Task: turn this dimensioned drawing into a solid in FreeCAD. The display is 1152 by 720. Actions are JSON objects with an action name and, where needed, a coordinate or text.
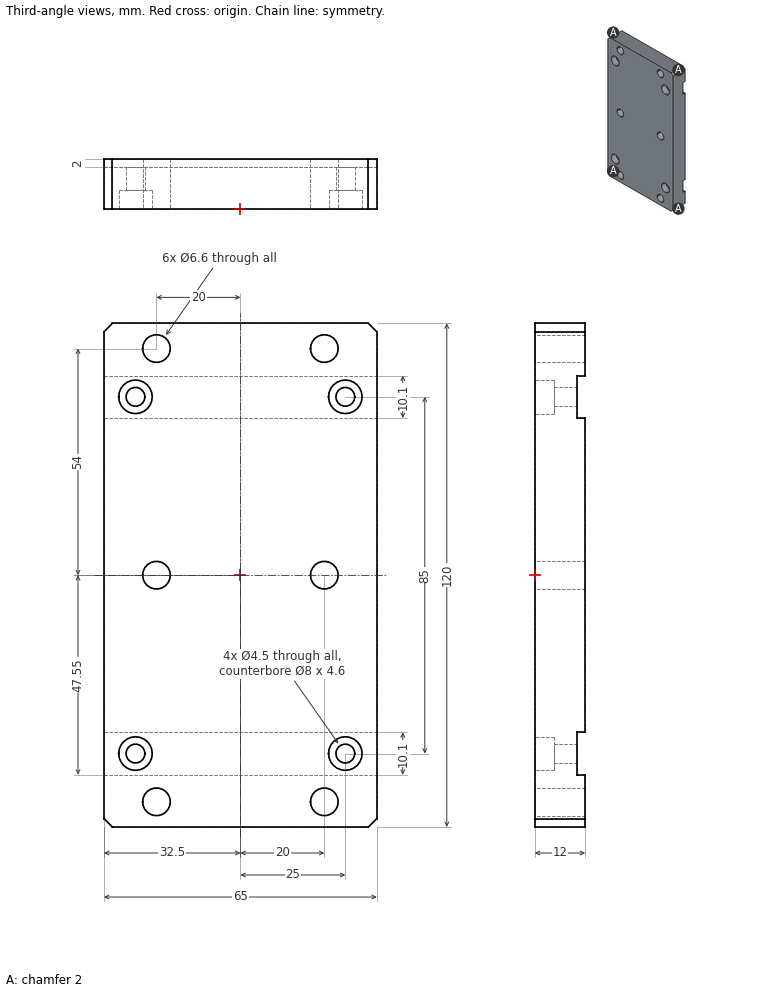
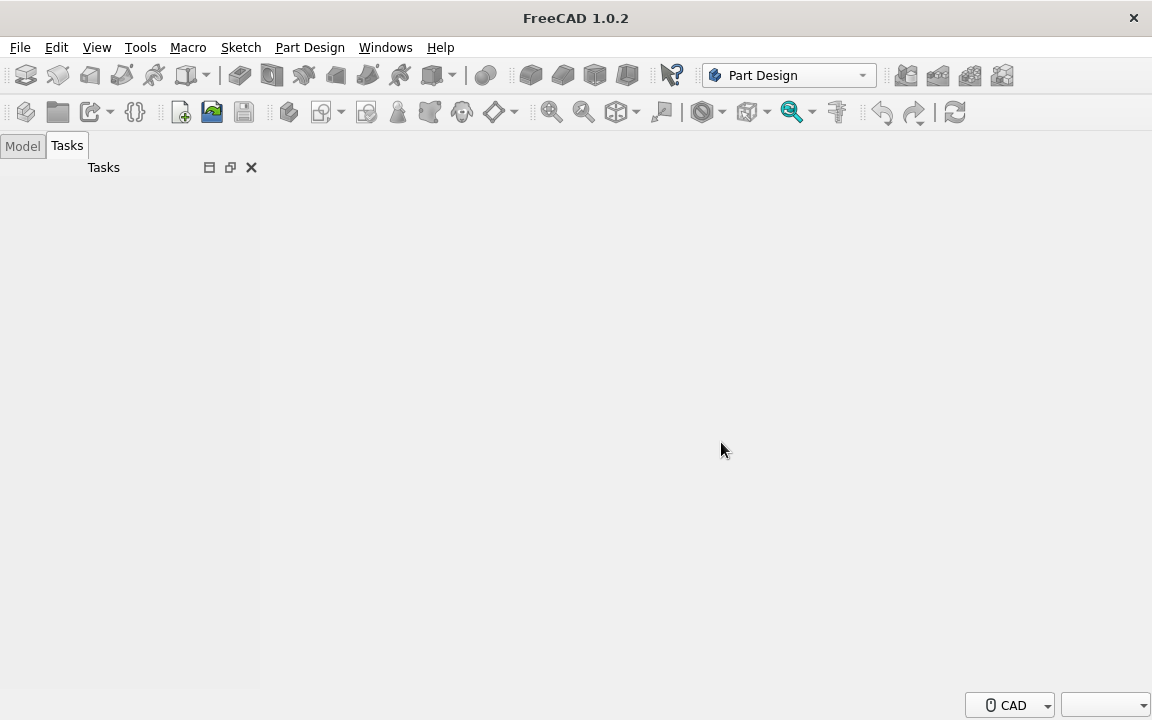
{"action": "key", "text": "ctrl+n"}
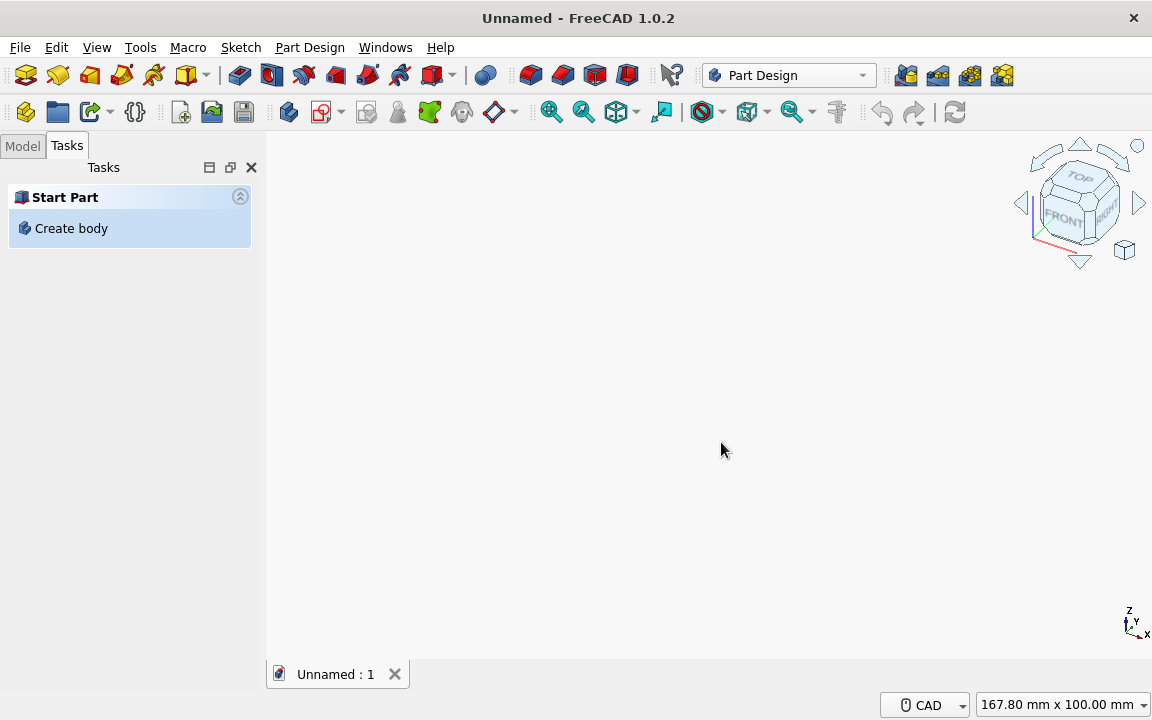
{"action": "left_click", "coordinate": [322, 112]}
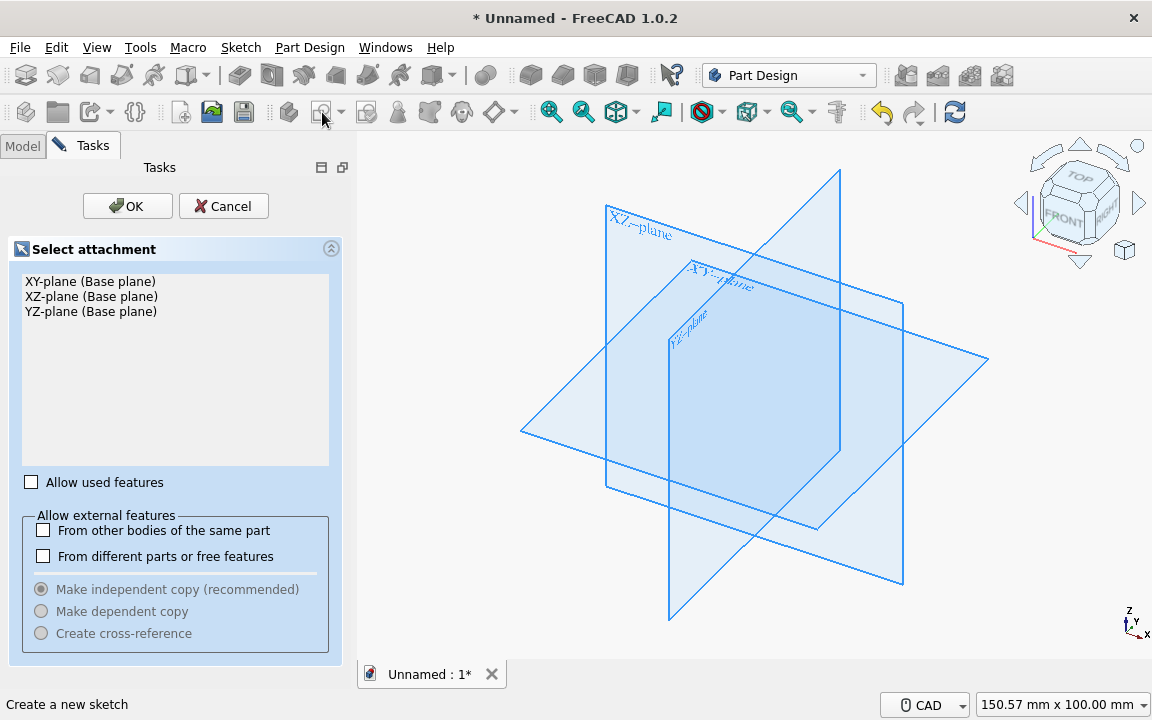
{"action": "left_click", "coordinate": [82, 296]}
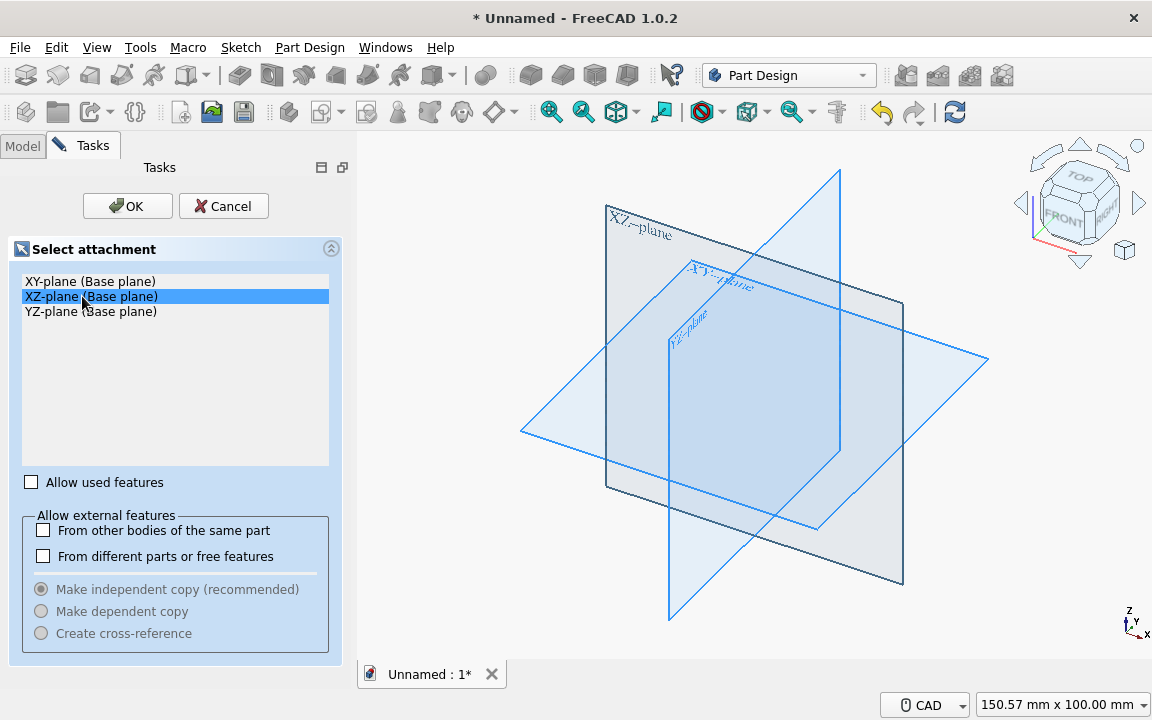
{"action": "left_click", "coordinate": [128, 206]}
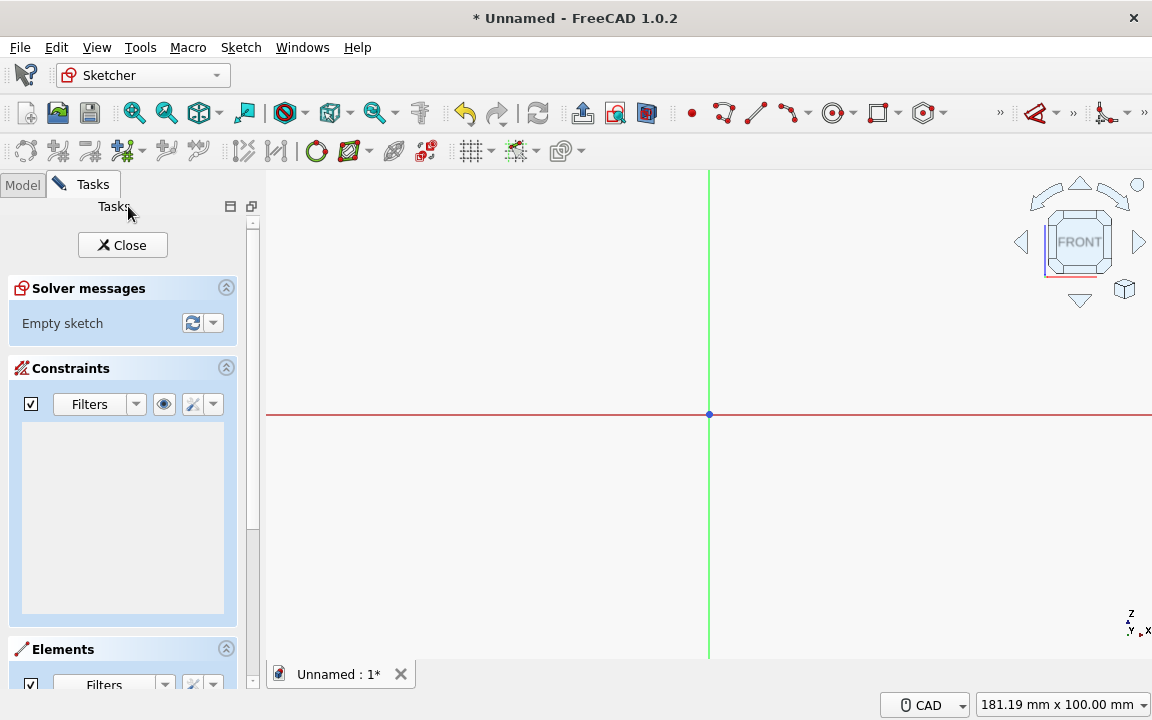
{"action": "scroll", "coordinate": [557, 414], "scroll_direction": "down", "scroll_amount": 3}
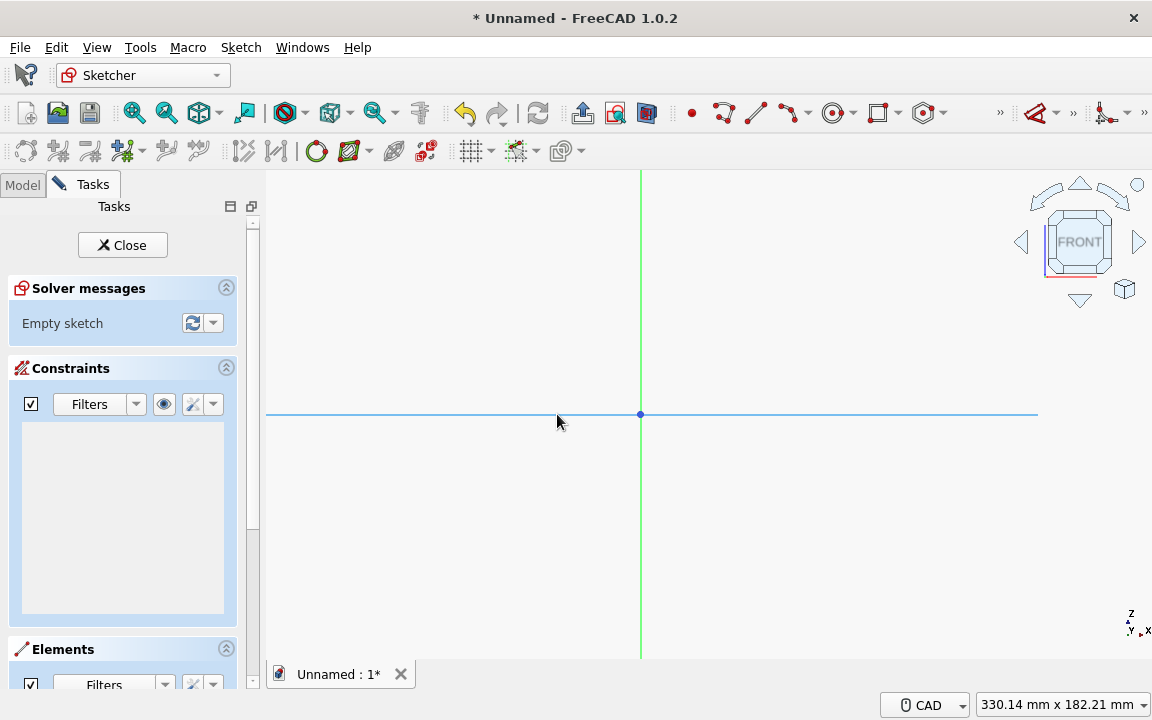
{"action": "left_click", "coordinate": [900, 114]}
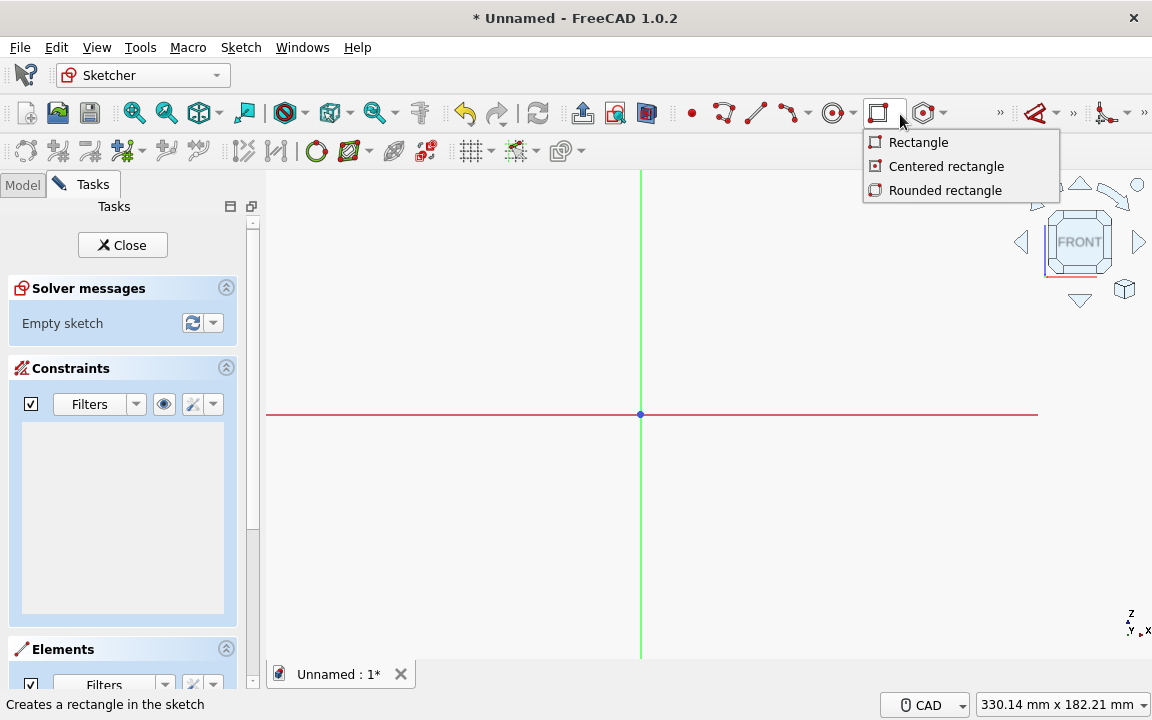
{"action": "left_click", "coordinate": [962, 166]}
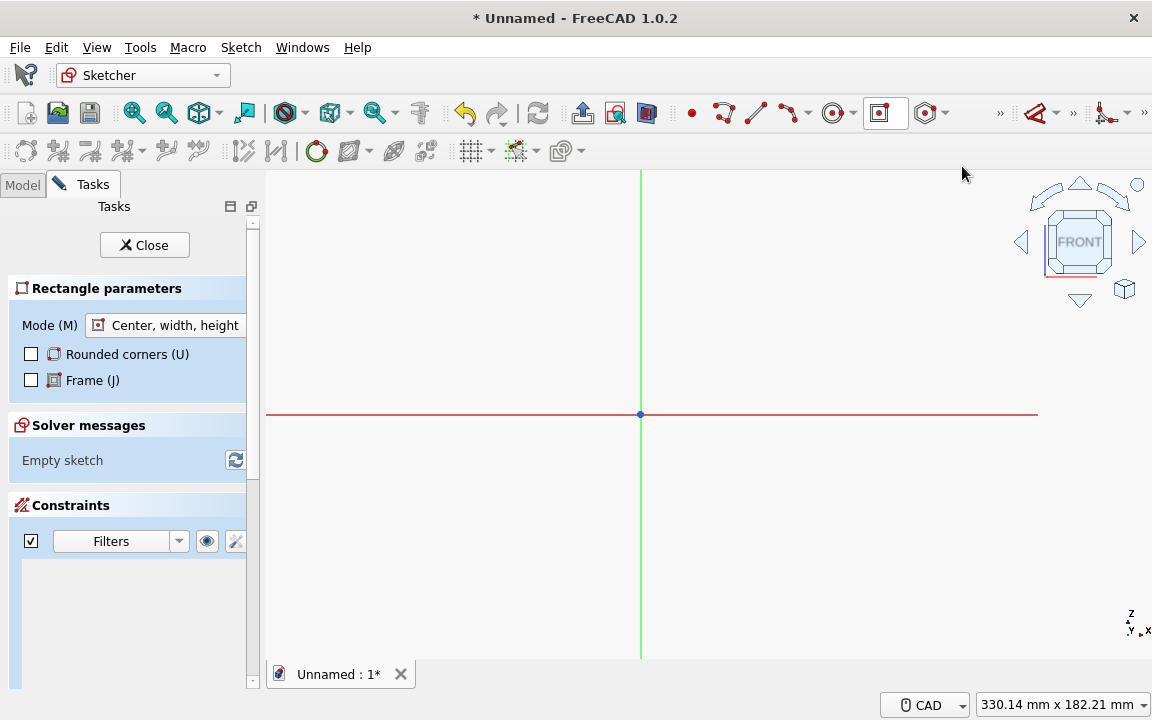
{"action": "left_click", "coordinate": [641, 414]}
{"action": "mouse_move", "coordinate": [728, 253]}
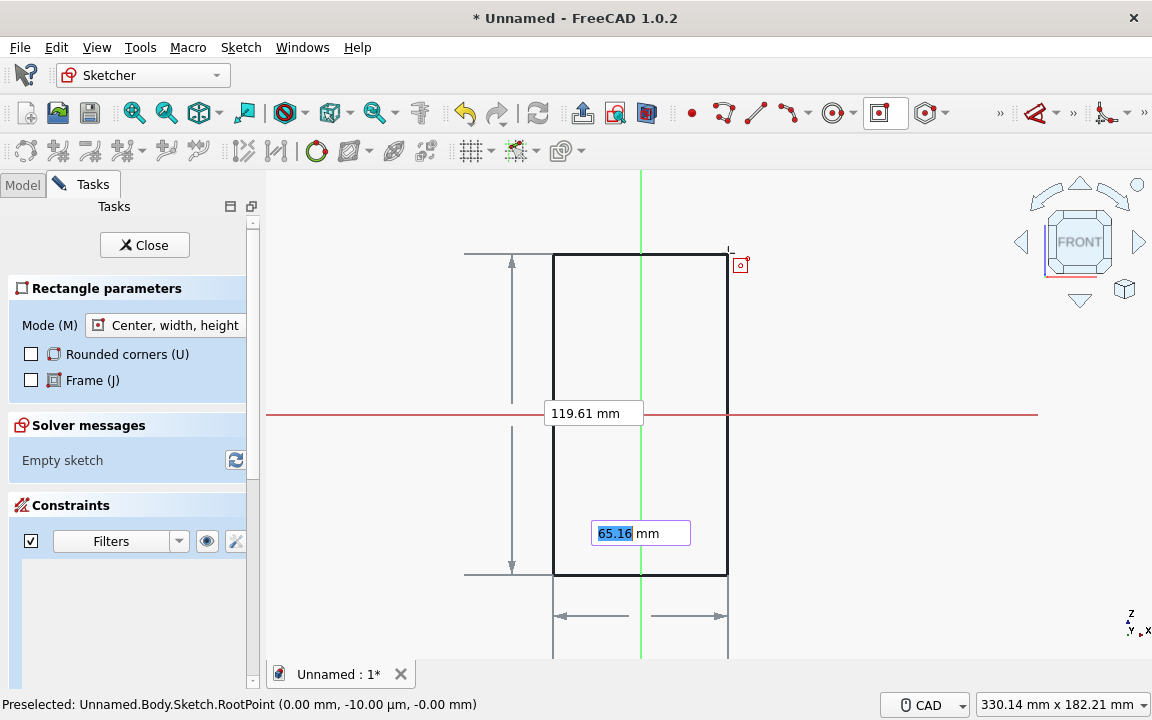
{"action": "type", "text": "65"}
{"action": "key", "text": "Tab"}
{"action": "type", "text": "120"}
{"action": "key", "text": "Return"}
{"action": "key", "text": "Escape"}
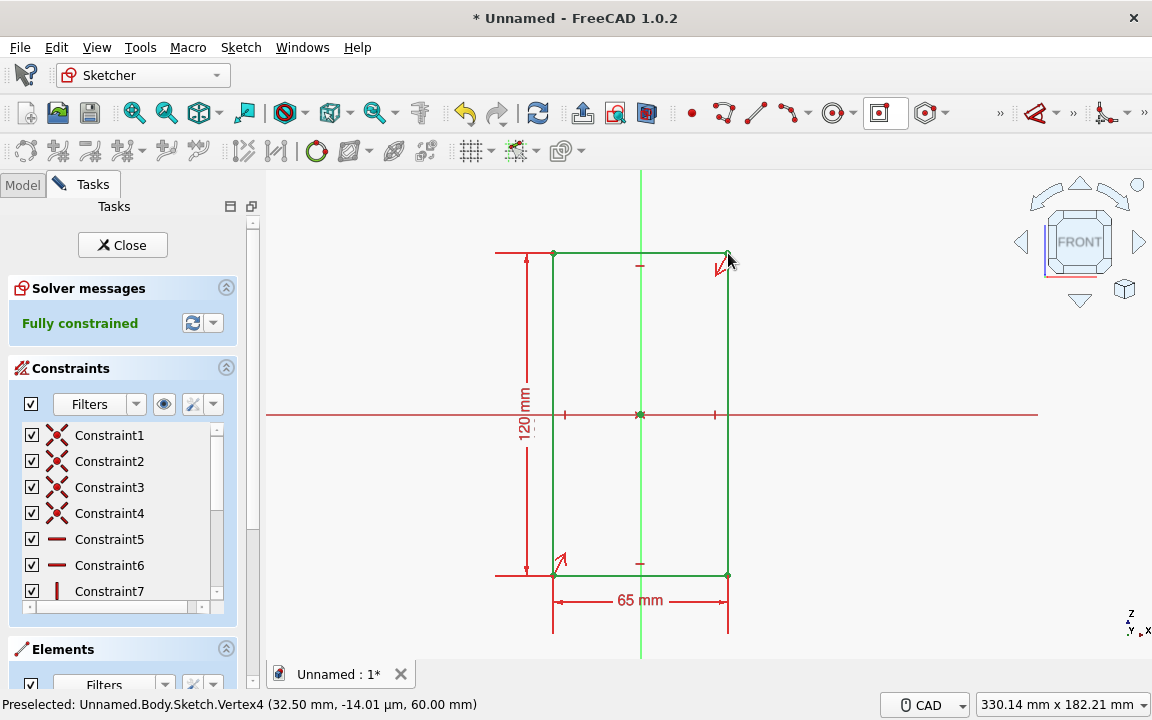
{"action": "left_click", "coordinate": [123, 245]}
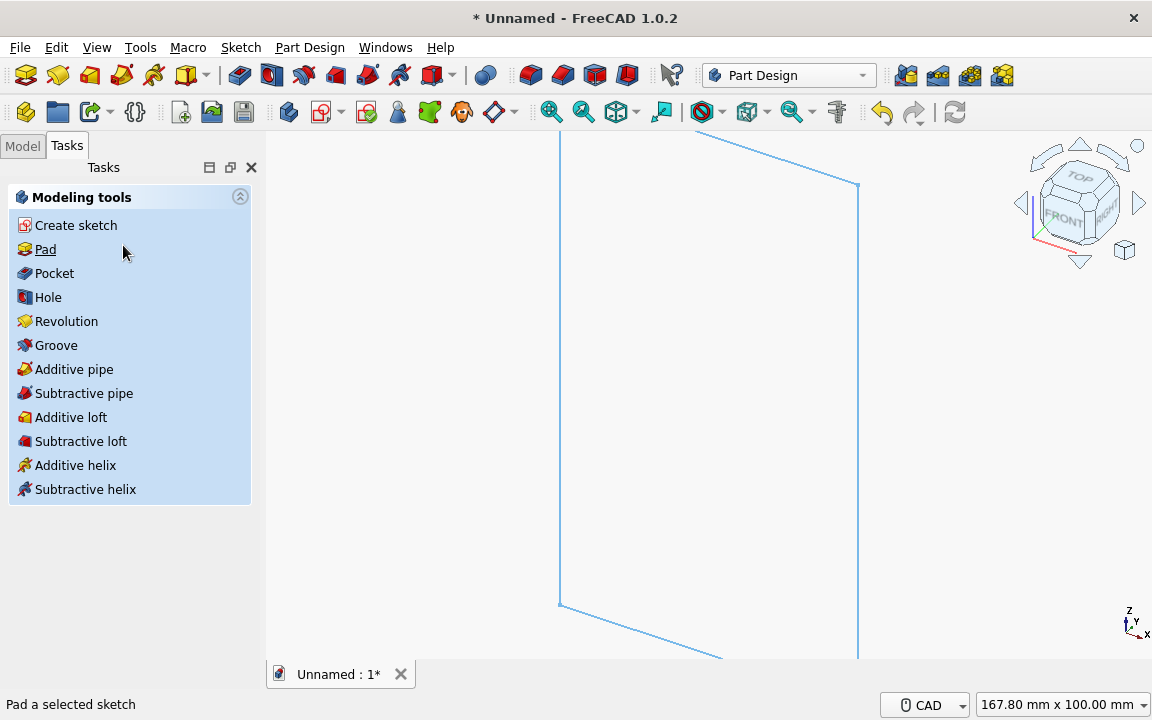
{"action": "left_click", "coordinate": [26, 76]}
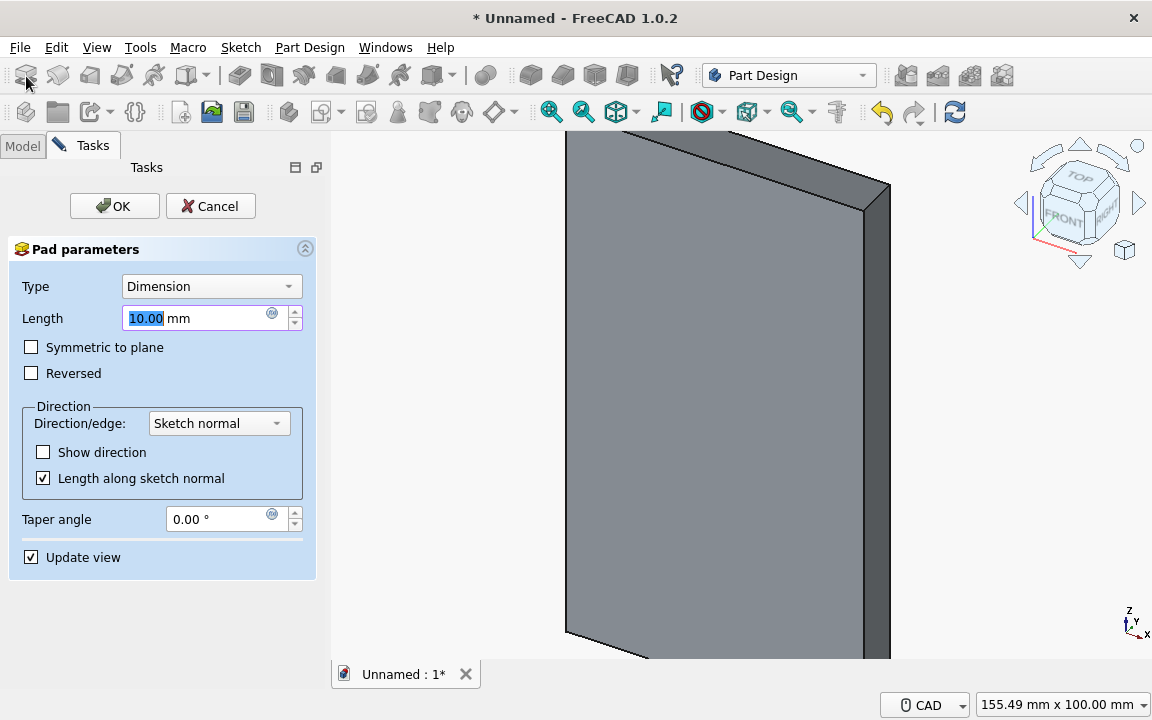
{"action": "type", "text": "12"}
{"action": "key", "text": "Tab"}